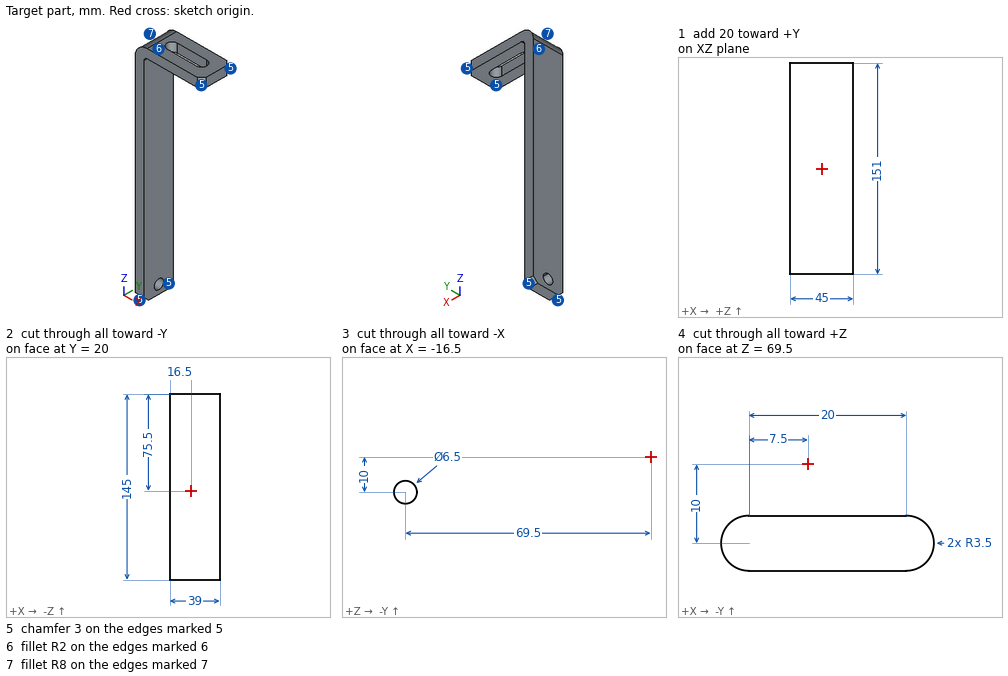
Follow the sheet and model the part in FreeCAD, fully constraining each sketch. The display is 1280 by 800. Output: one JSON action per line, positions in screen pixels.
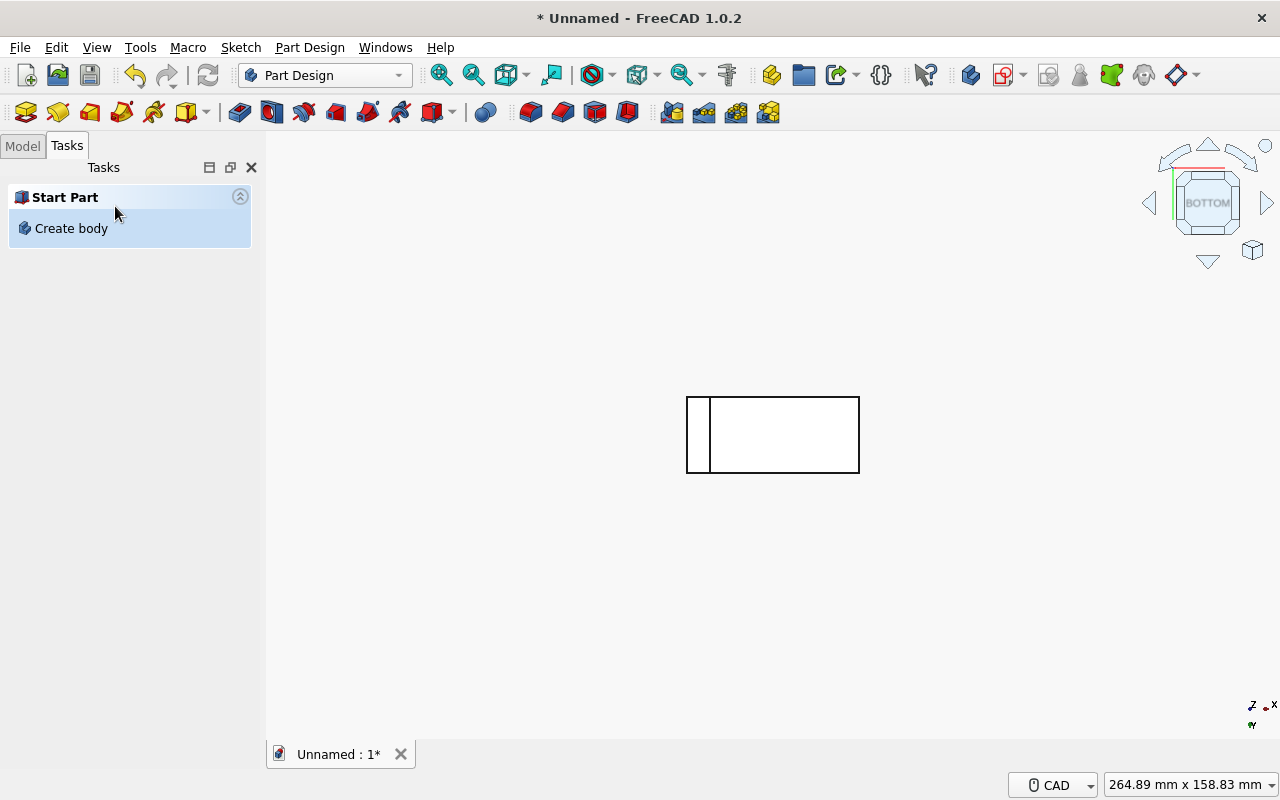
{"action": "left_click", "coordinate": [442, 76]}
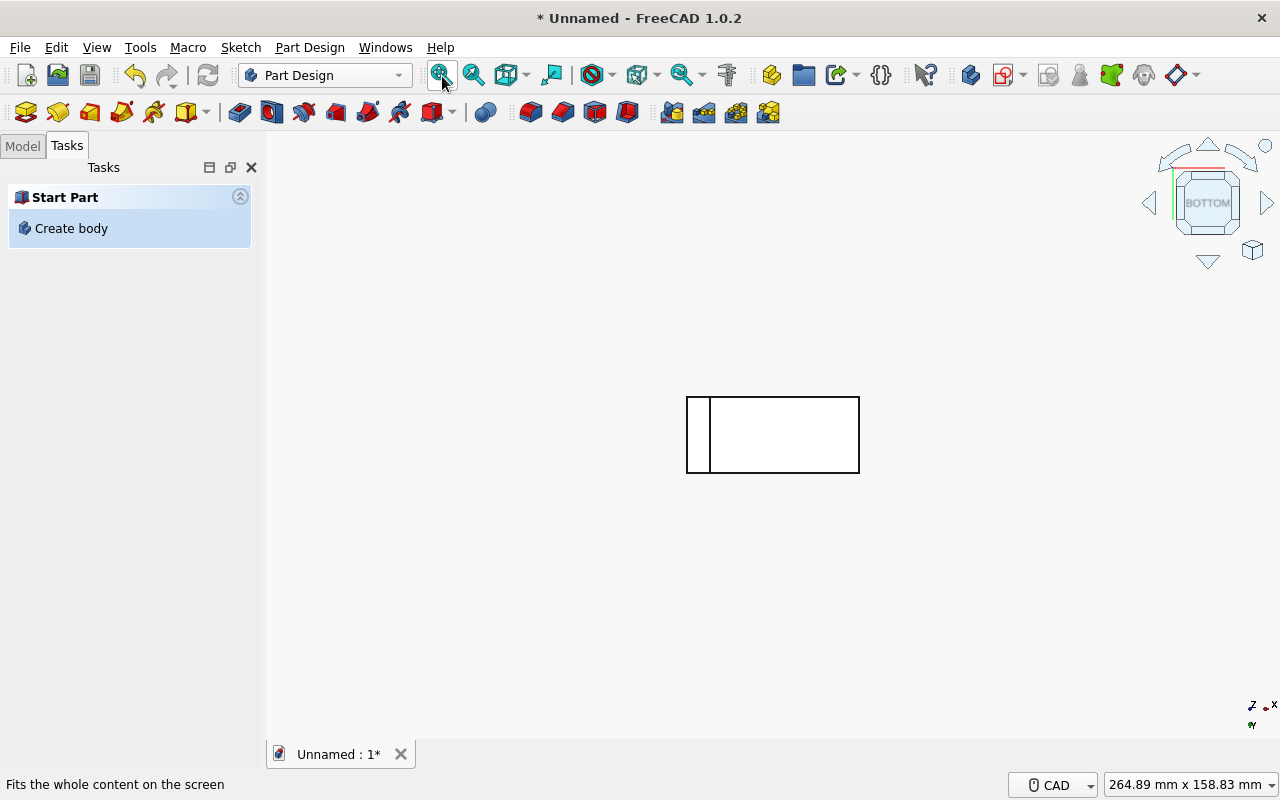
{"action": "left_click", "coordinate": [806, 434]}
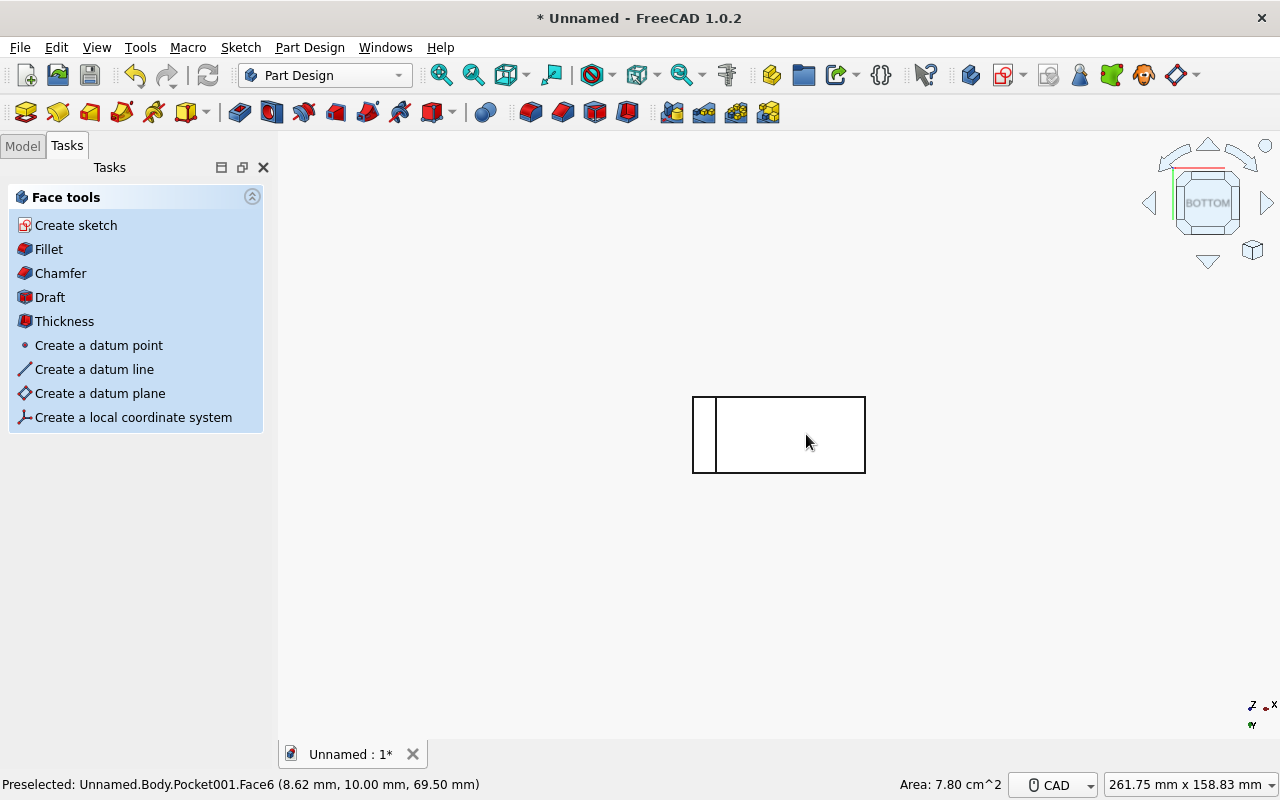
{"action": "left_click", "coordinate": [1004, 76]}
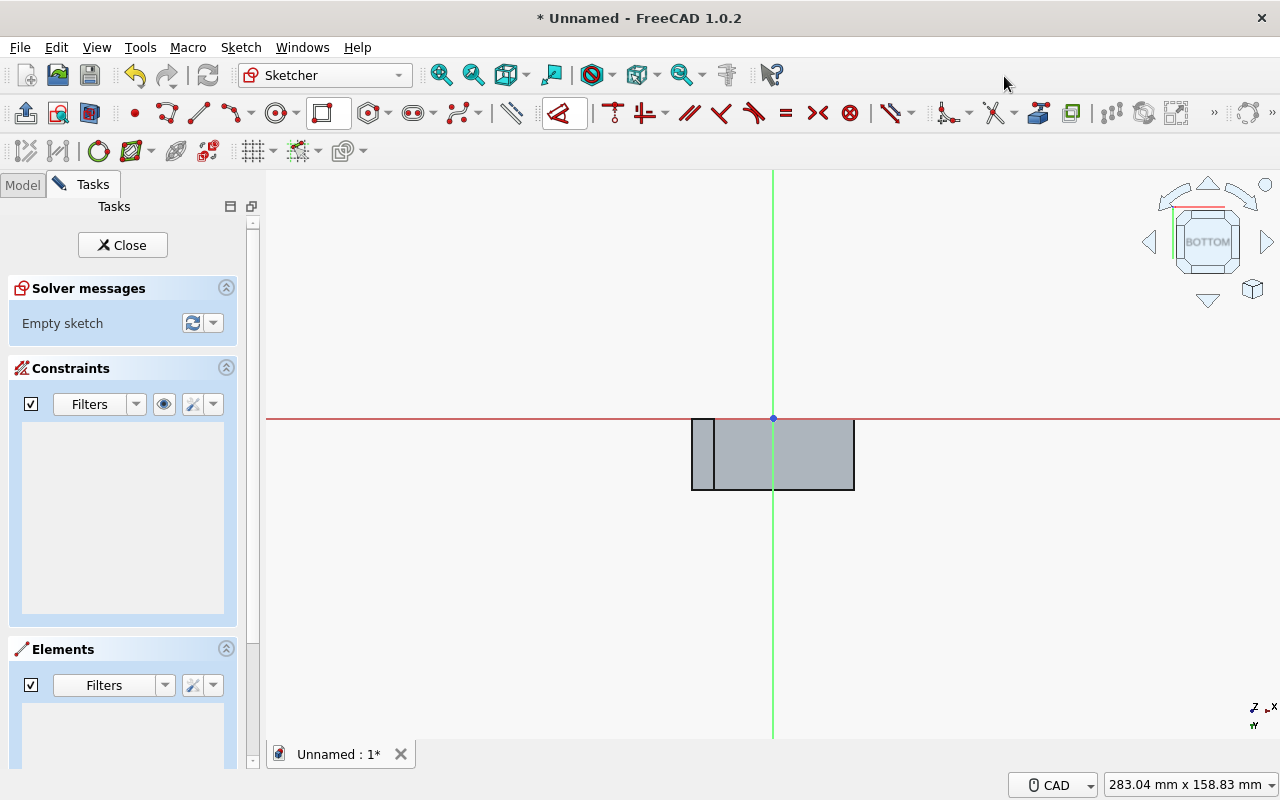
{"action": "left_click", "coordinate": [90, 114]}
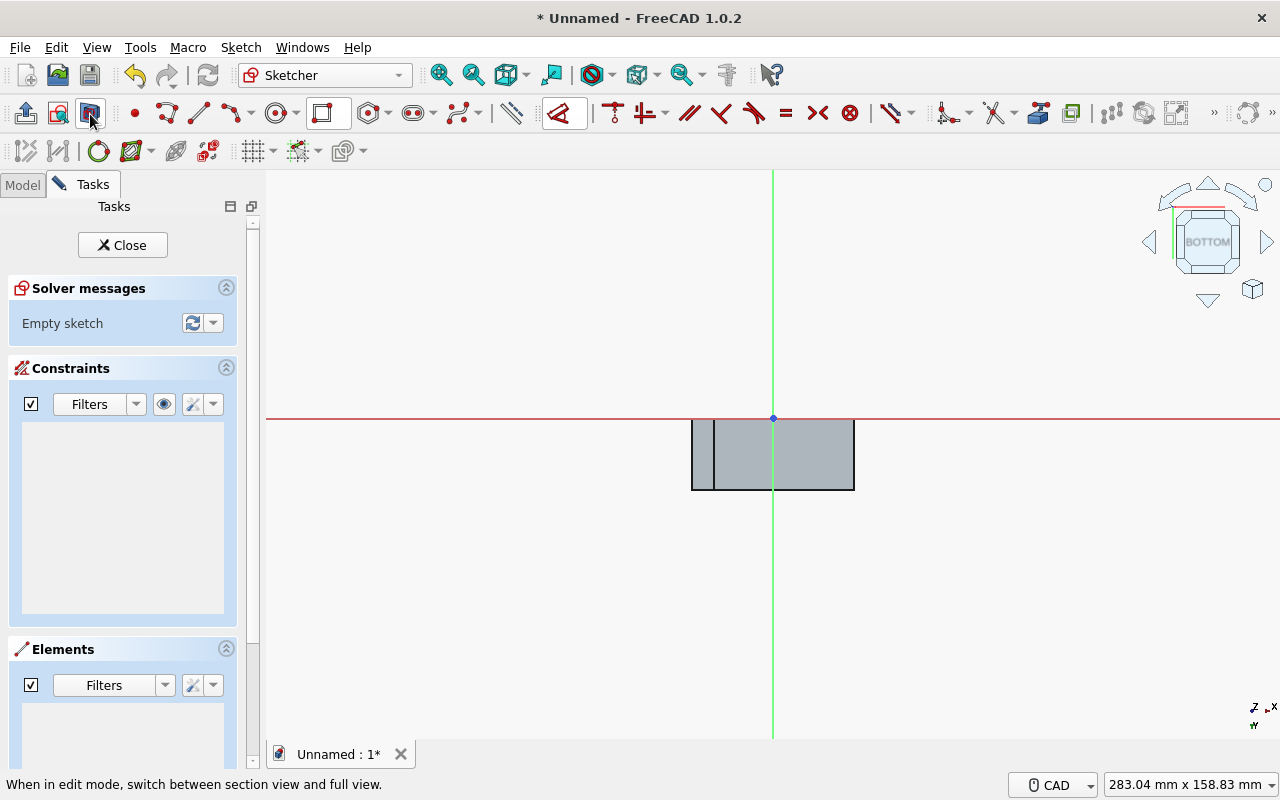
{"action": "scroll", "coordinate": [797, 441], "scroll_direction": "up", "scroll_amount": 9}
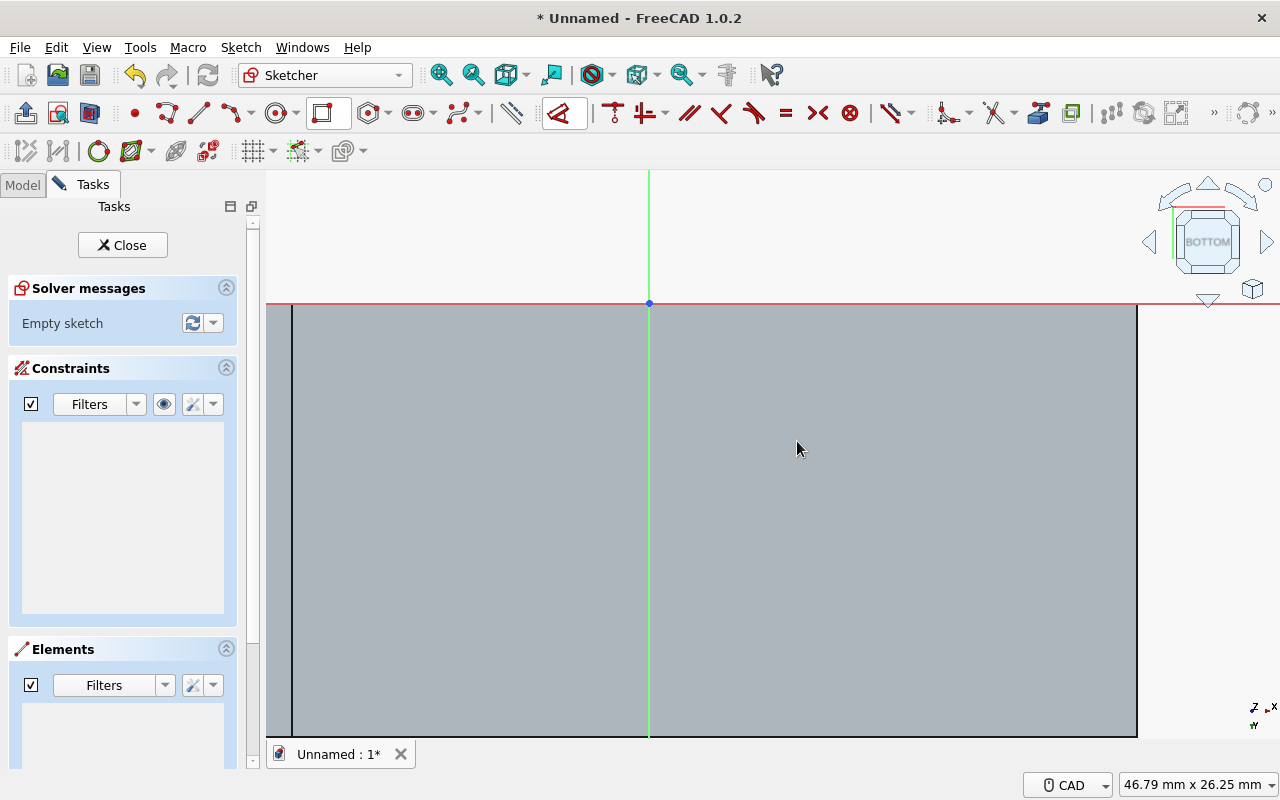
{"action": "left_click", "coordinate": [414, 114]}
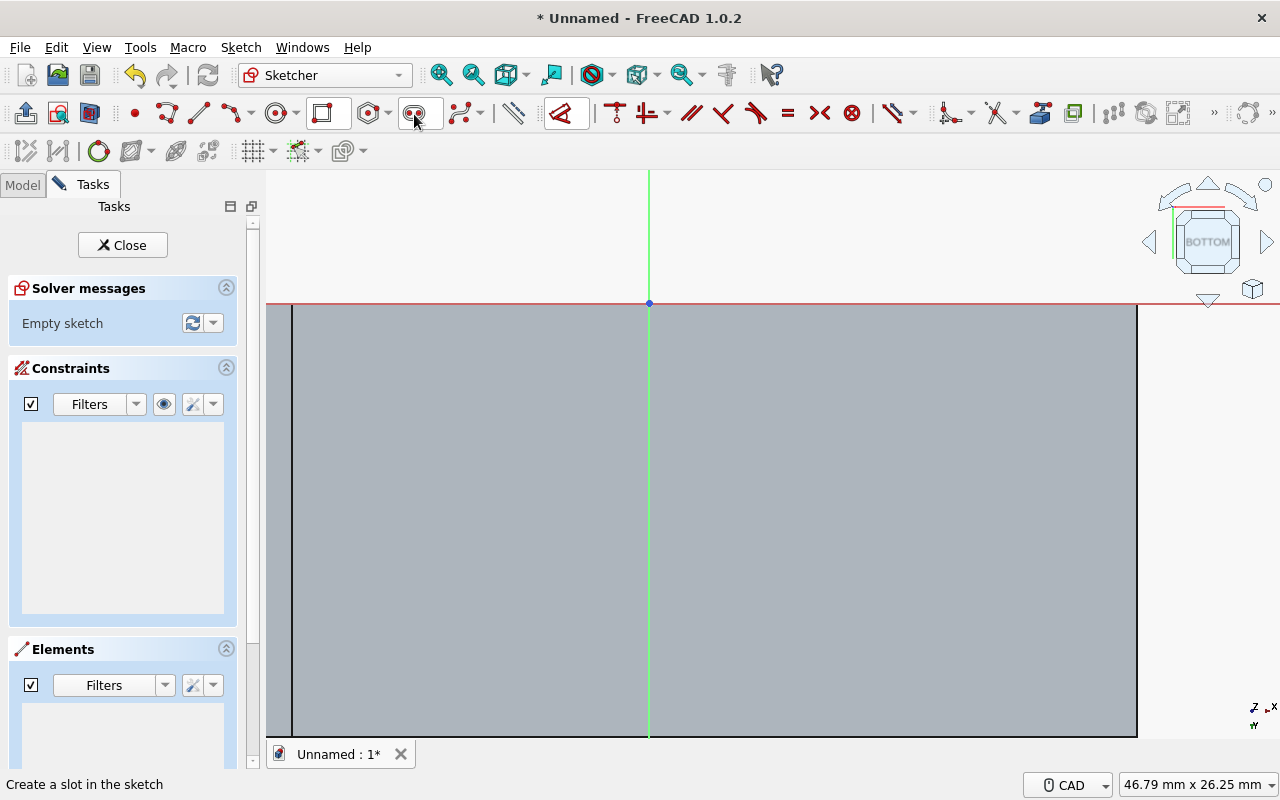
{"action": "left_click", "coordinate": [487, 520]}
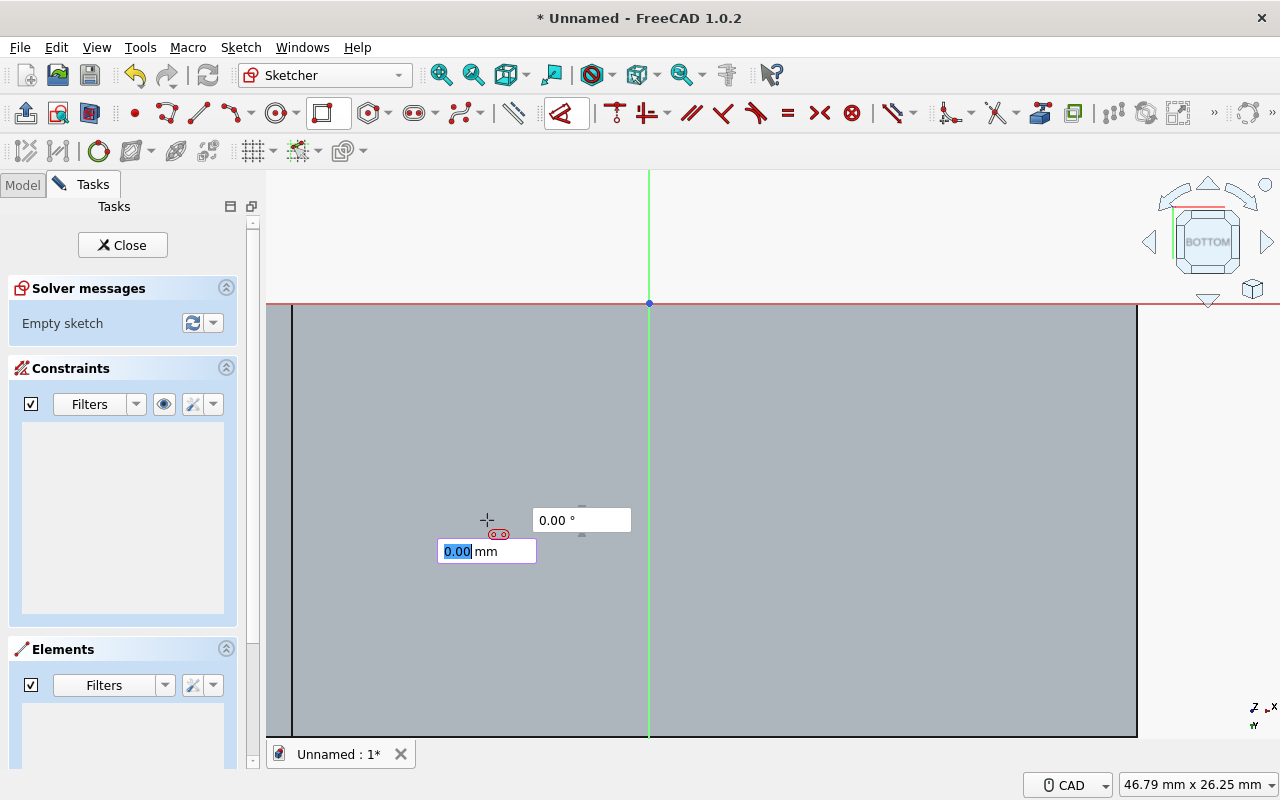
{"action": "left_click", "coordinate": [920, 520]}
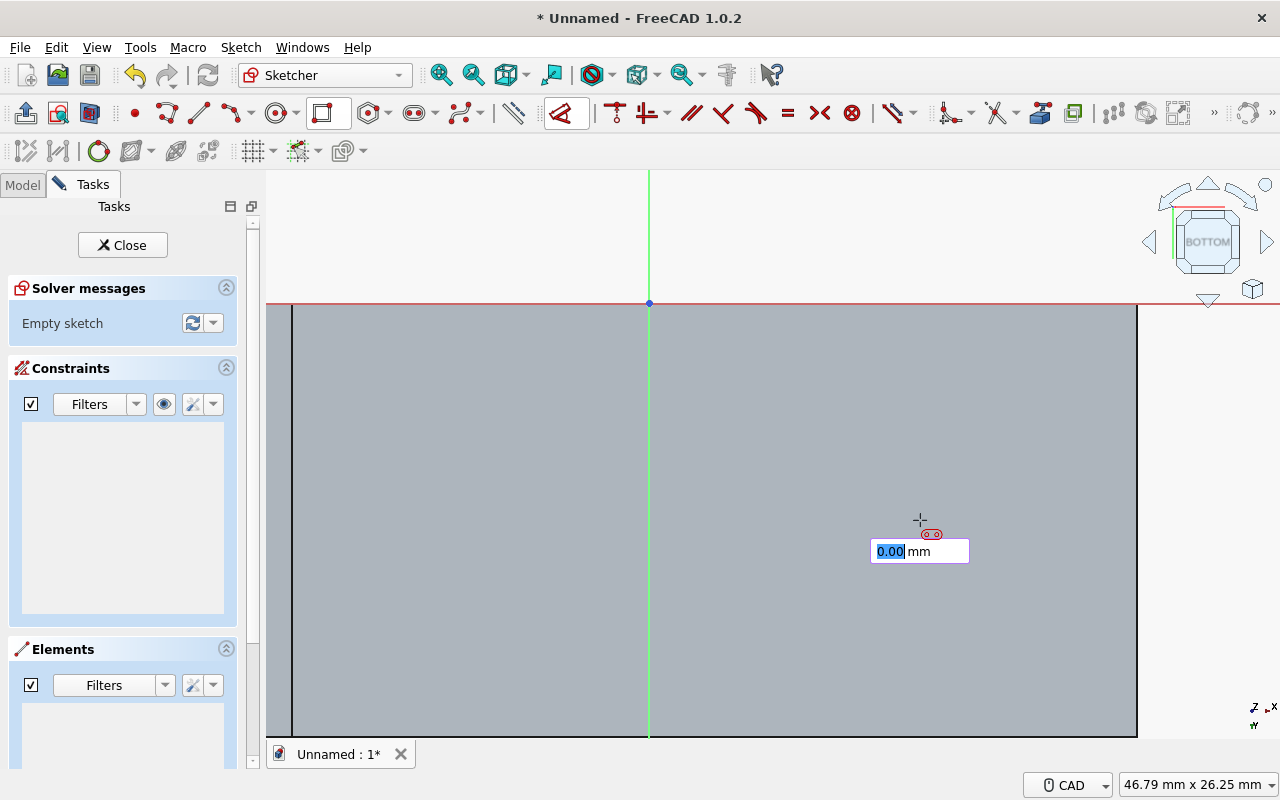
{"action": "left_click", "coordinate": [703, 596]}
{"action": "key", "text": "Escape"}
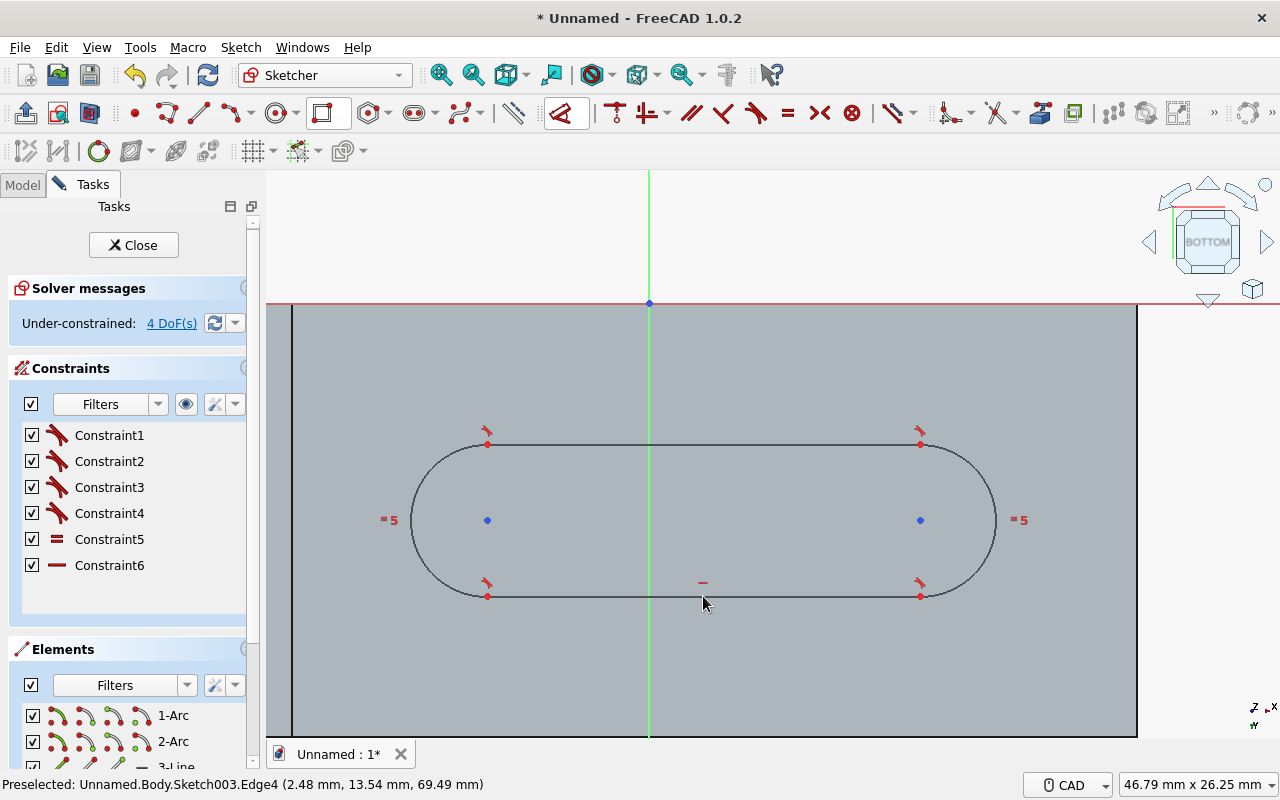
{"action": "left_click", "coordinate": [426, 476]}